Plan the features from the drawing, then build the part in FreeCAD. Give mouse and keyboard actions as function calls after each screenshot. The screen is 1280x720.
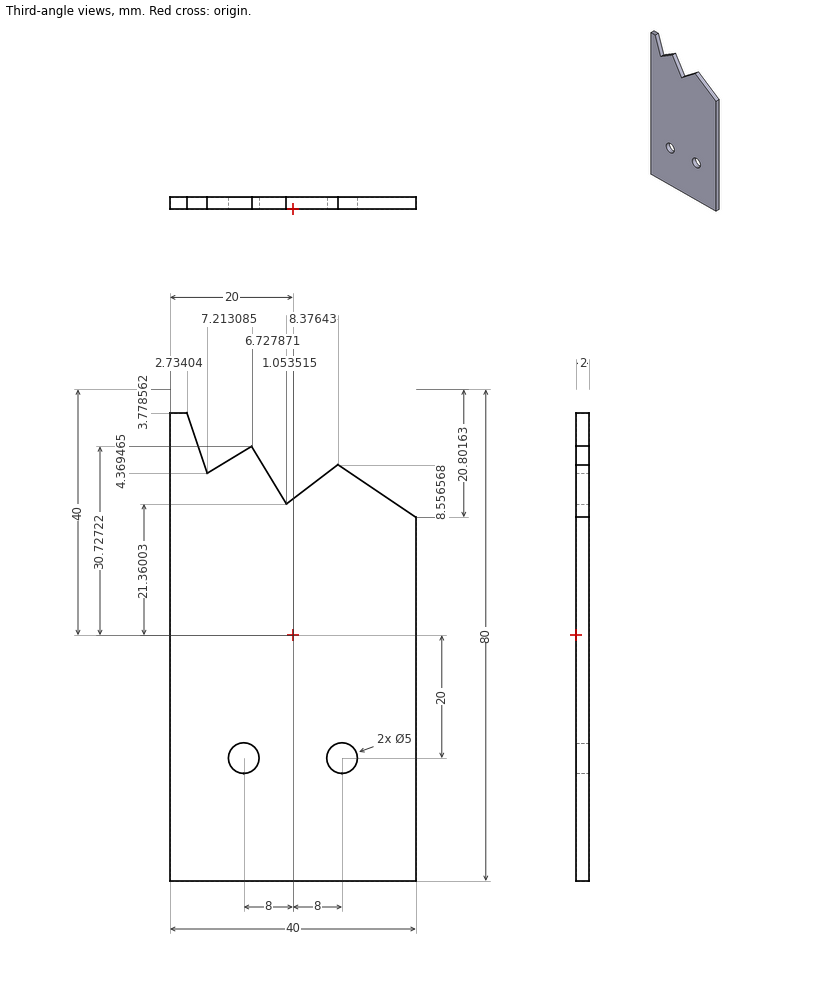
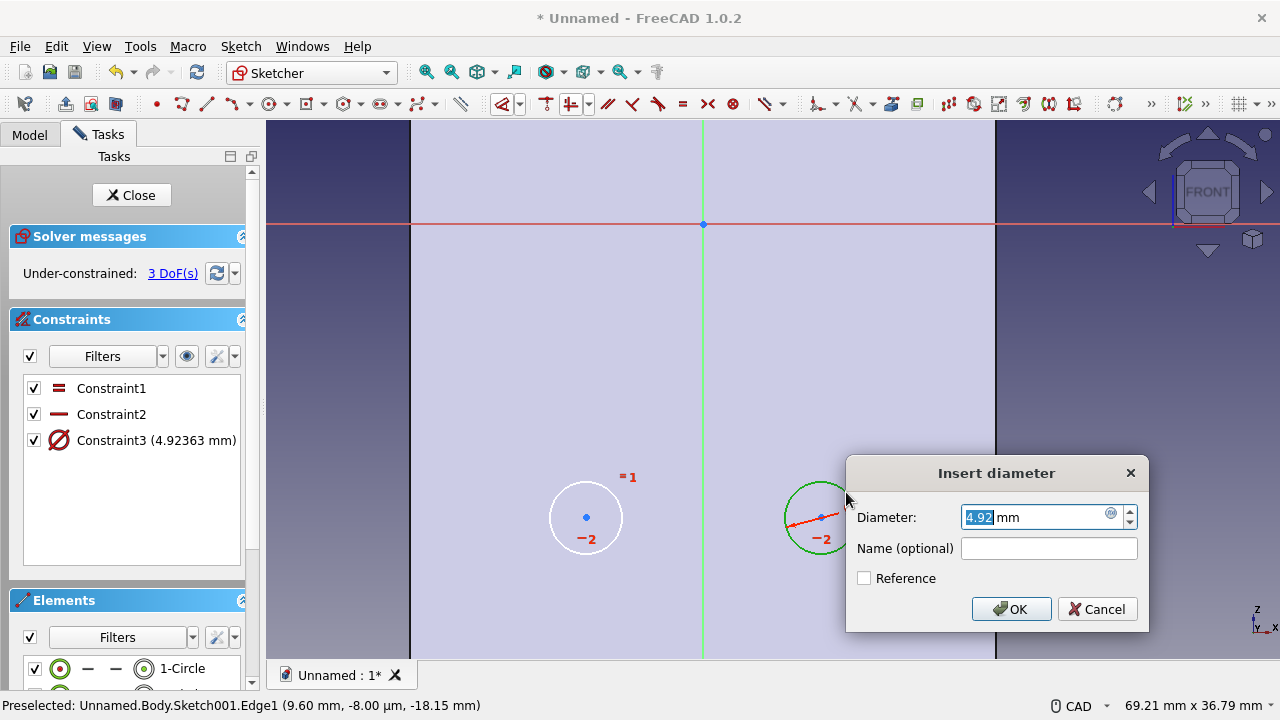
text(5)
key(Return)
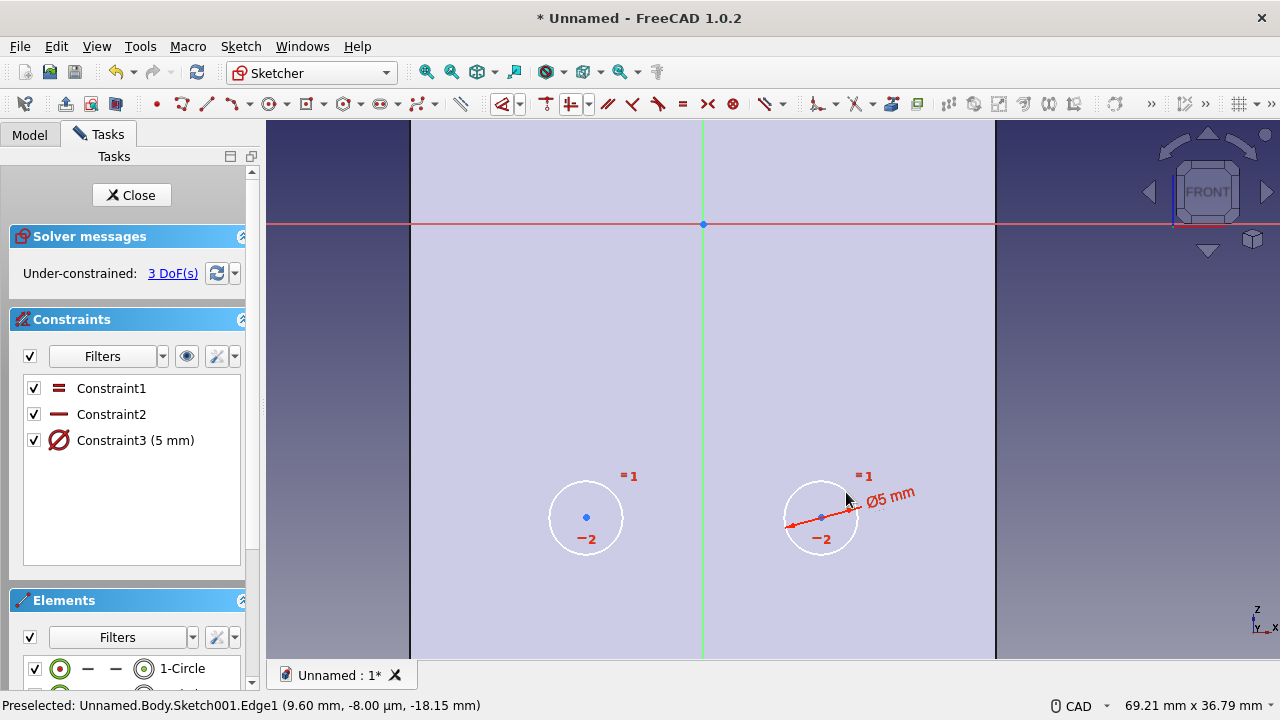
click(821, 518)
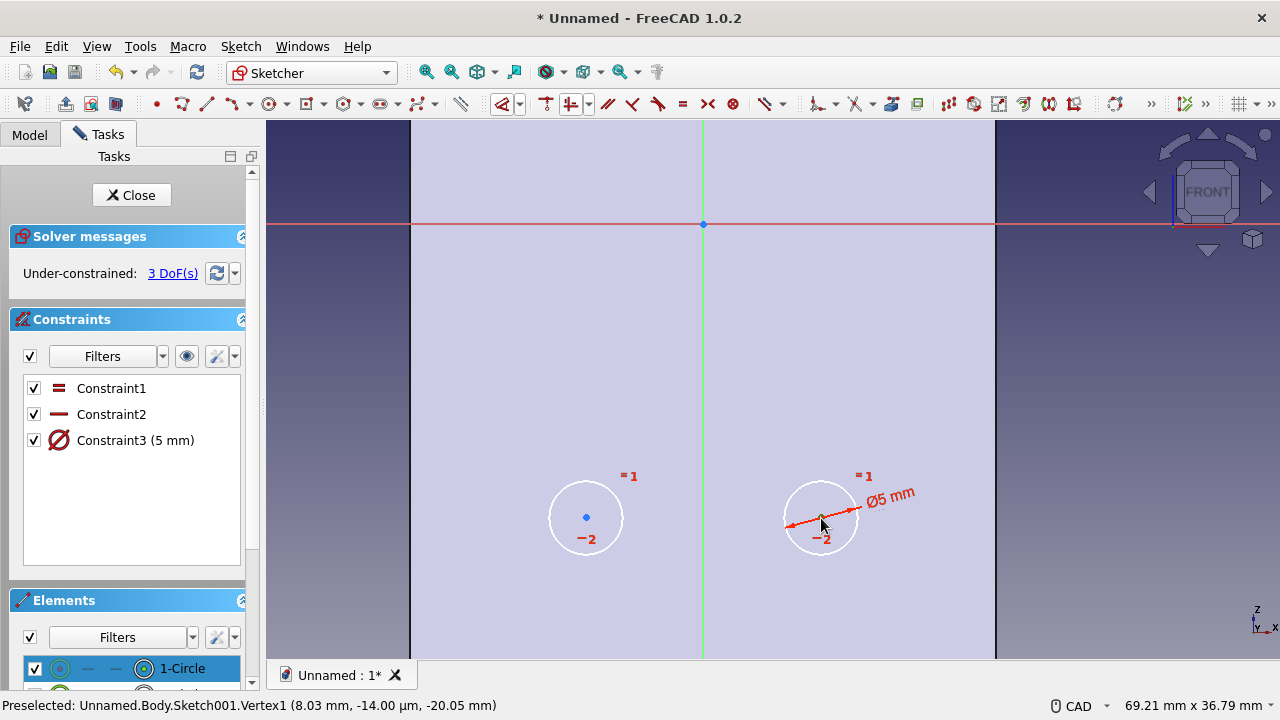
click(520, 104)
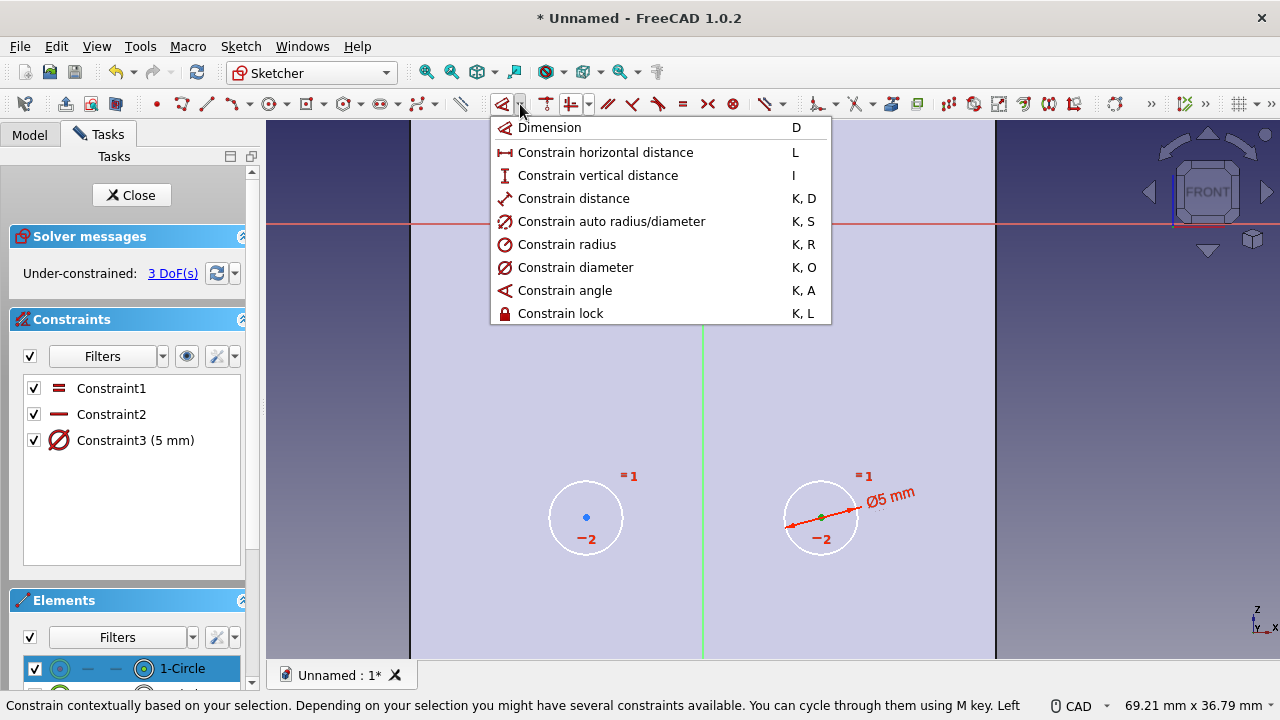
click(661, 152)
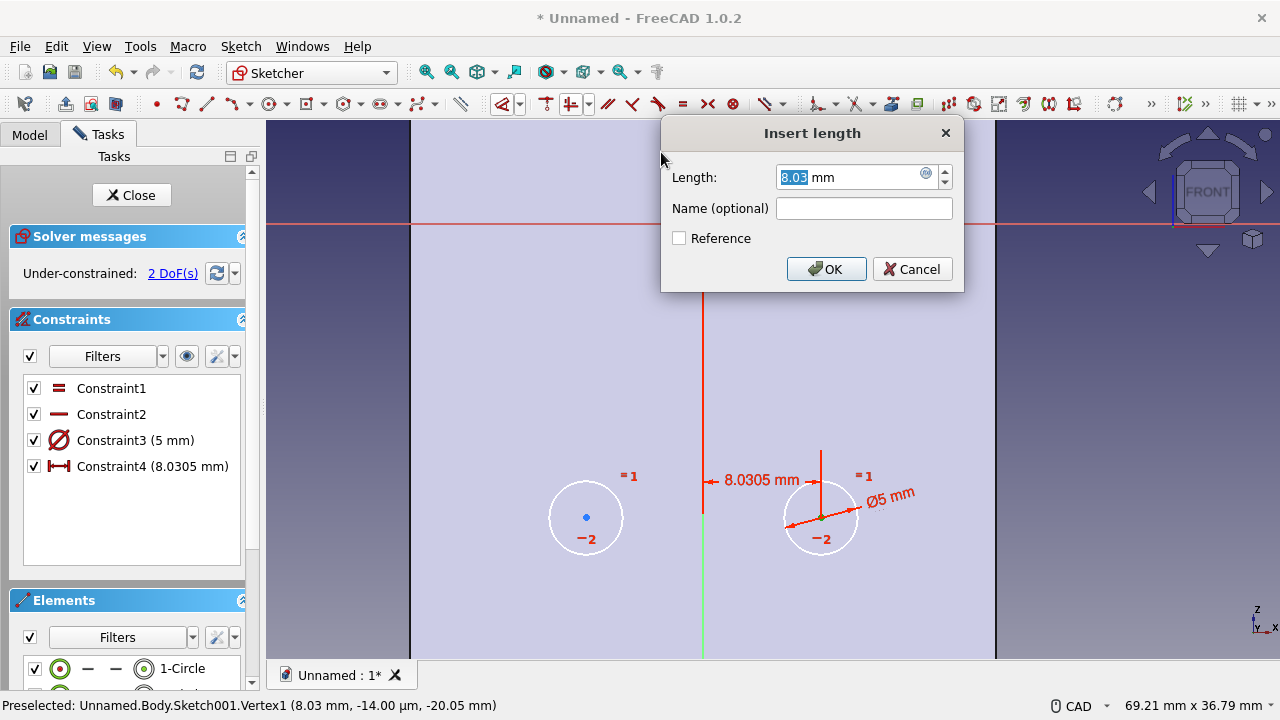
text(8)
key(Return)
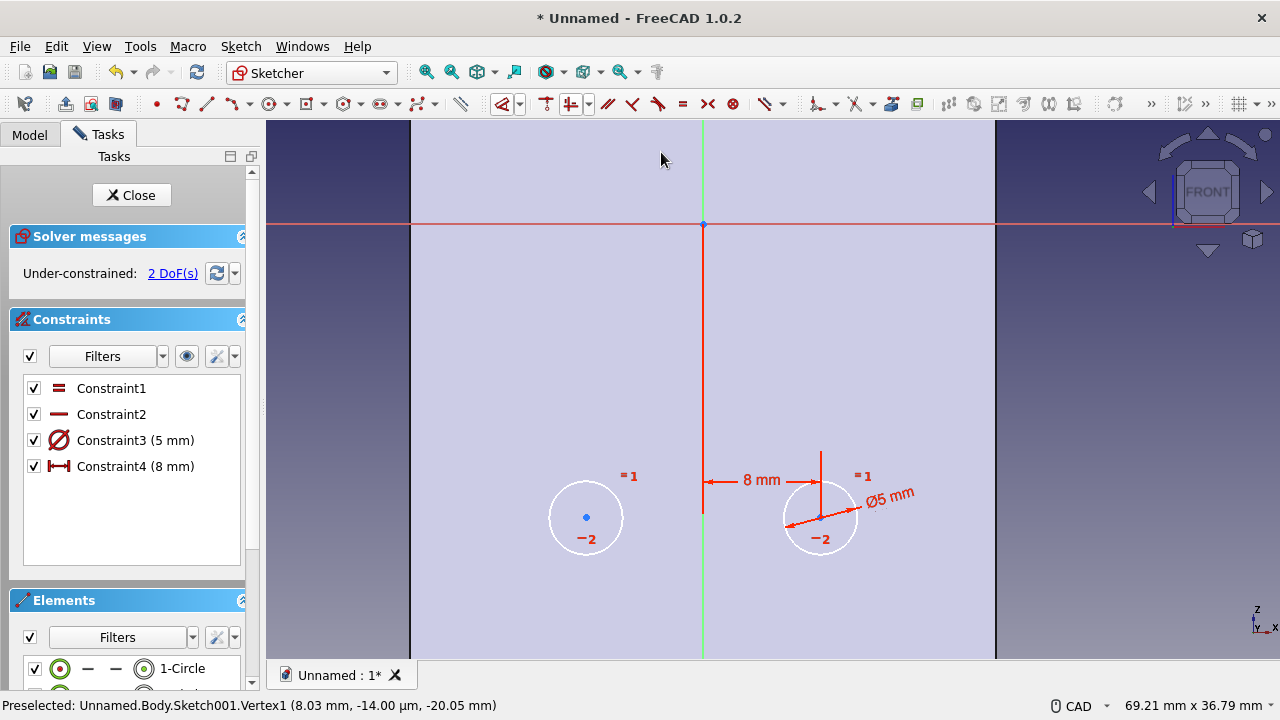
click(586, 518)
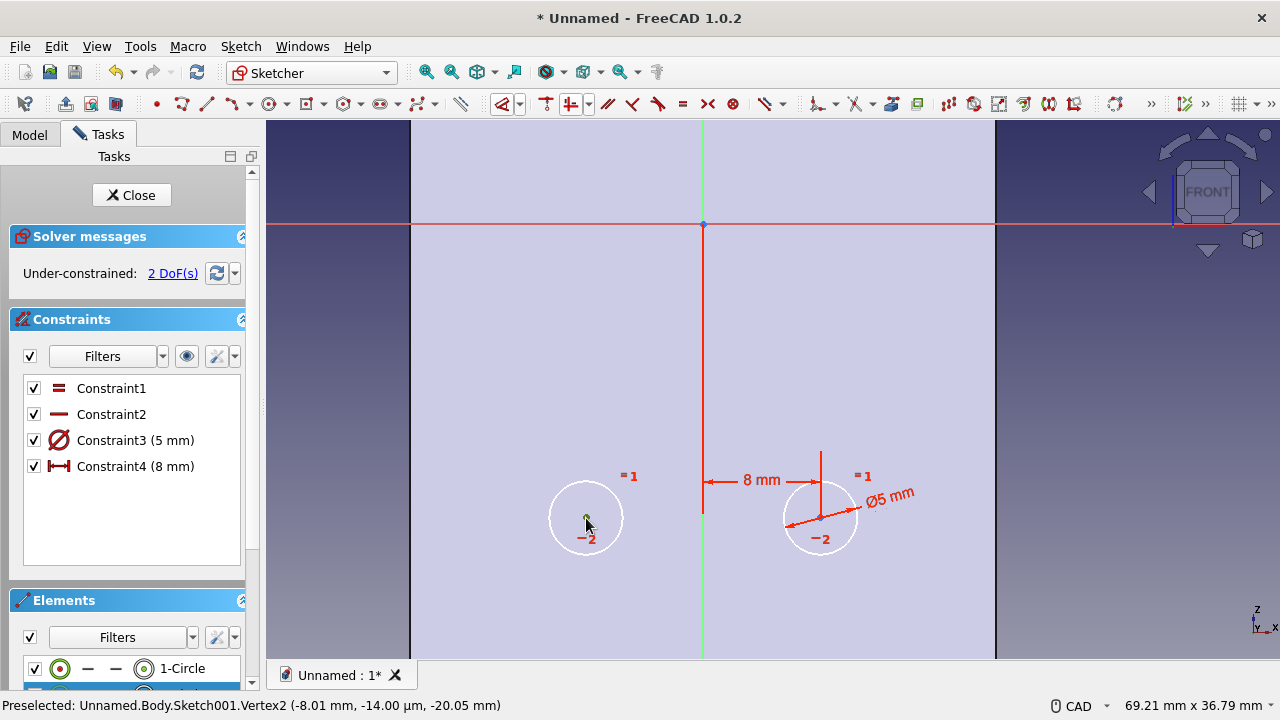
key(l)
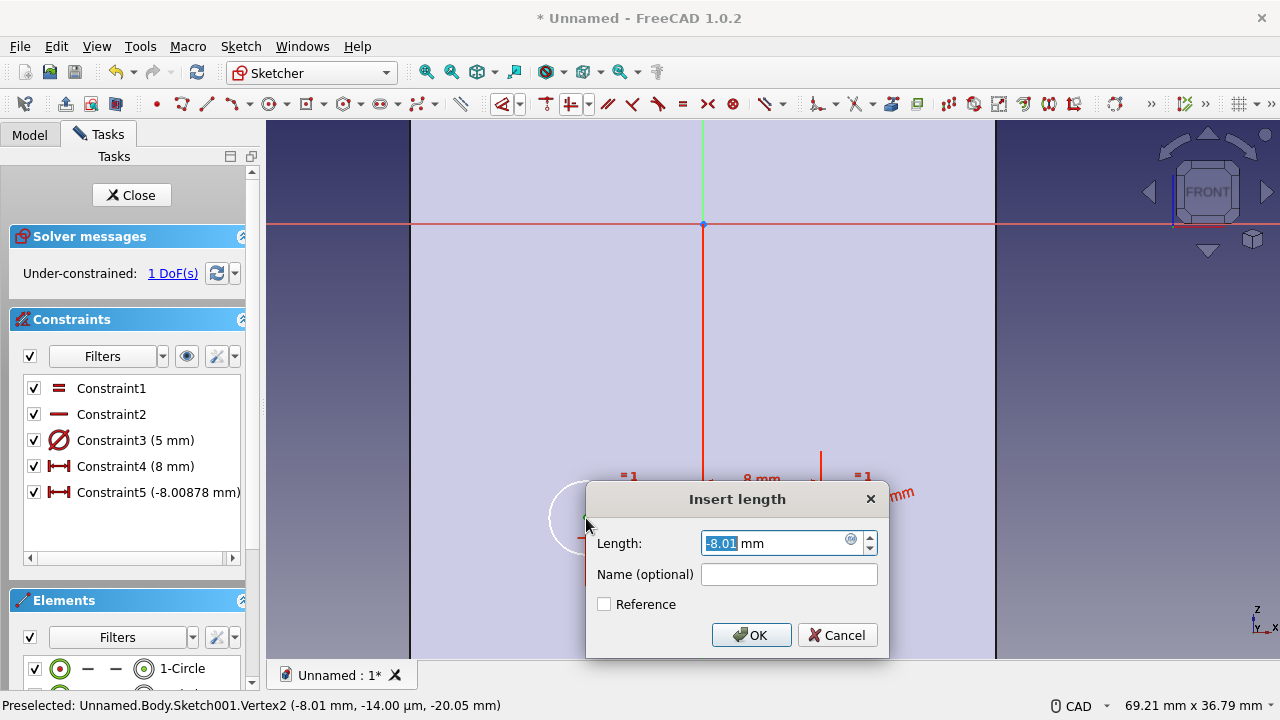
text(-8)
key(Return)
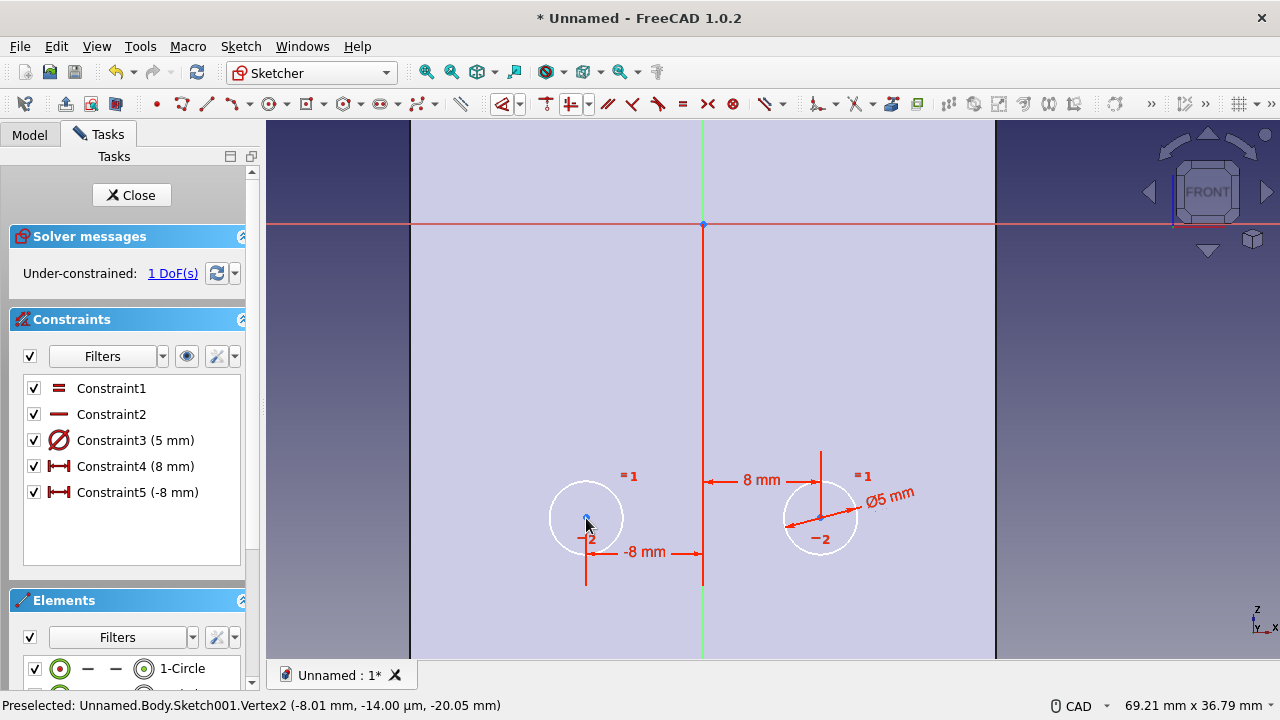
click(821, 518)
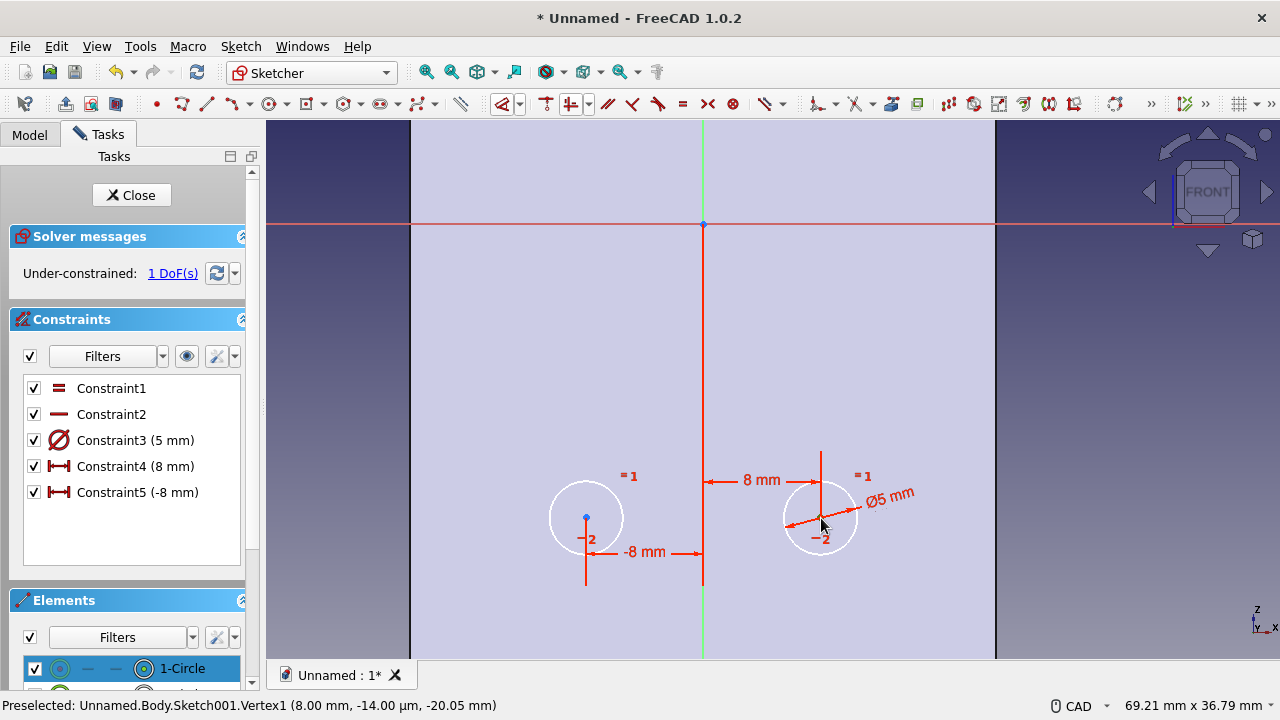
key(i)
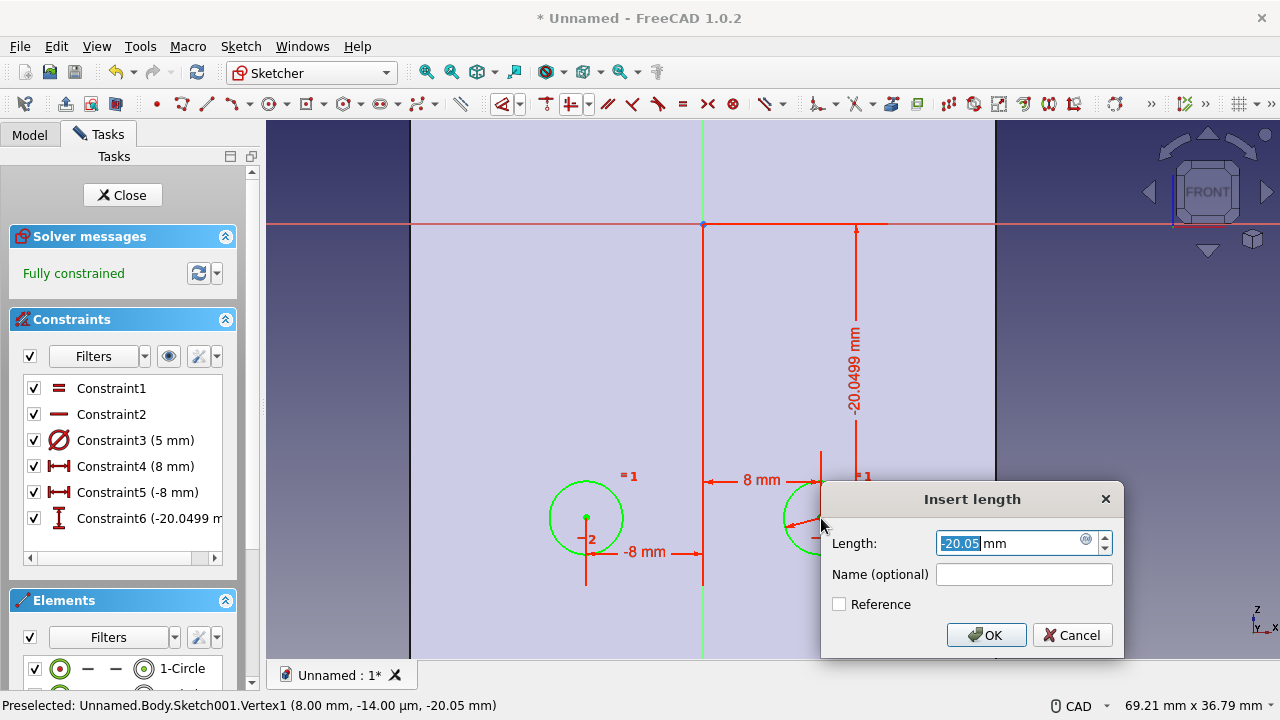
text(-20)
key(Return)